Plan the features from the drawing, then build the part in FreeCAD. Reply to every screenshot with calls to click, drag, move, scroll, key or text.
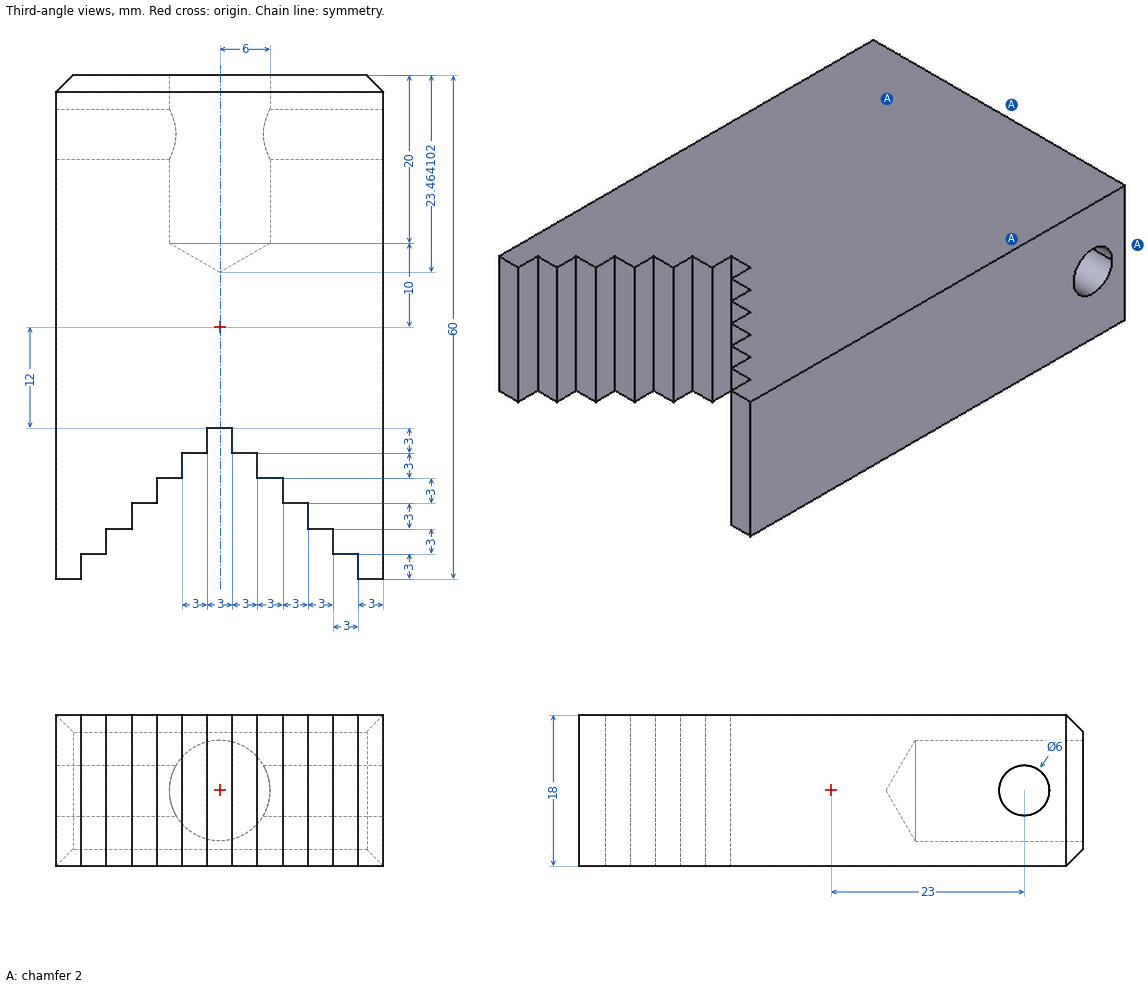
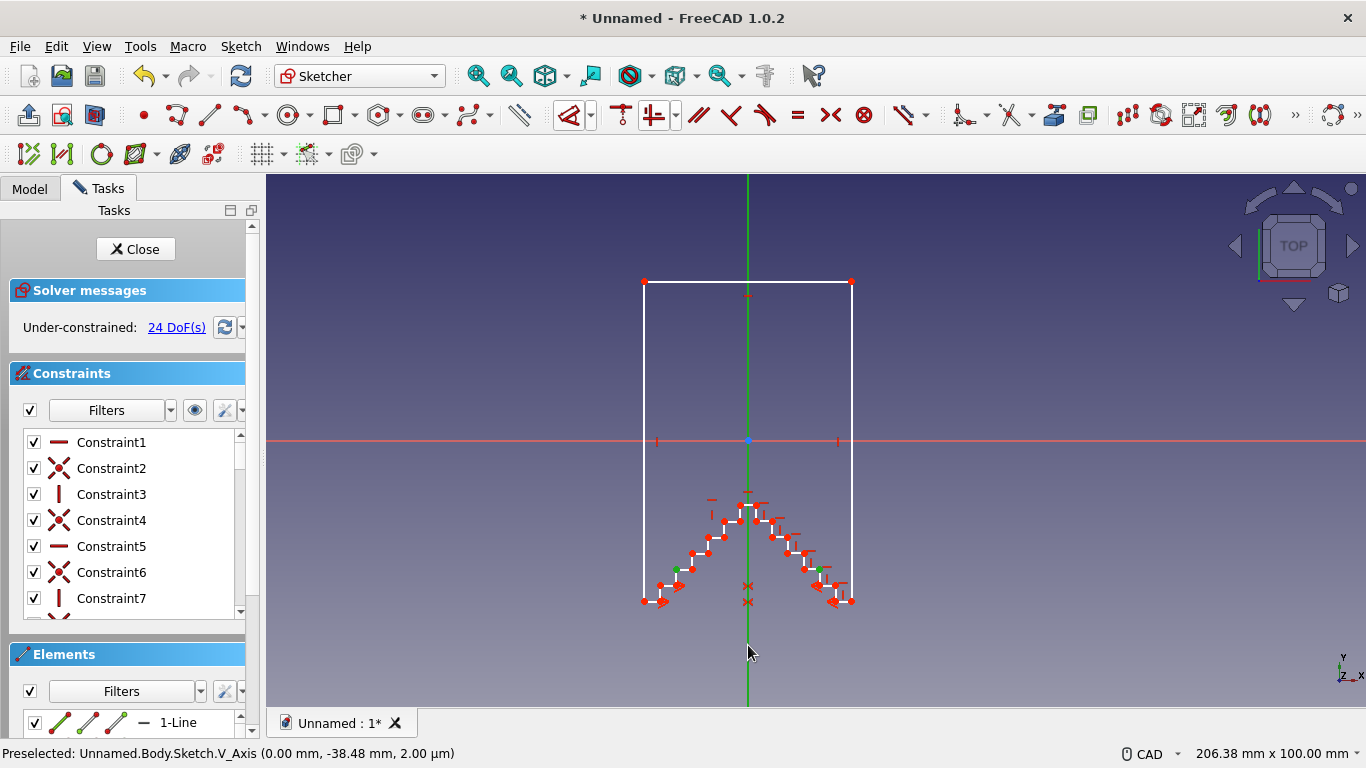
click(831, 116)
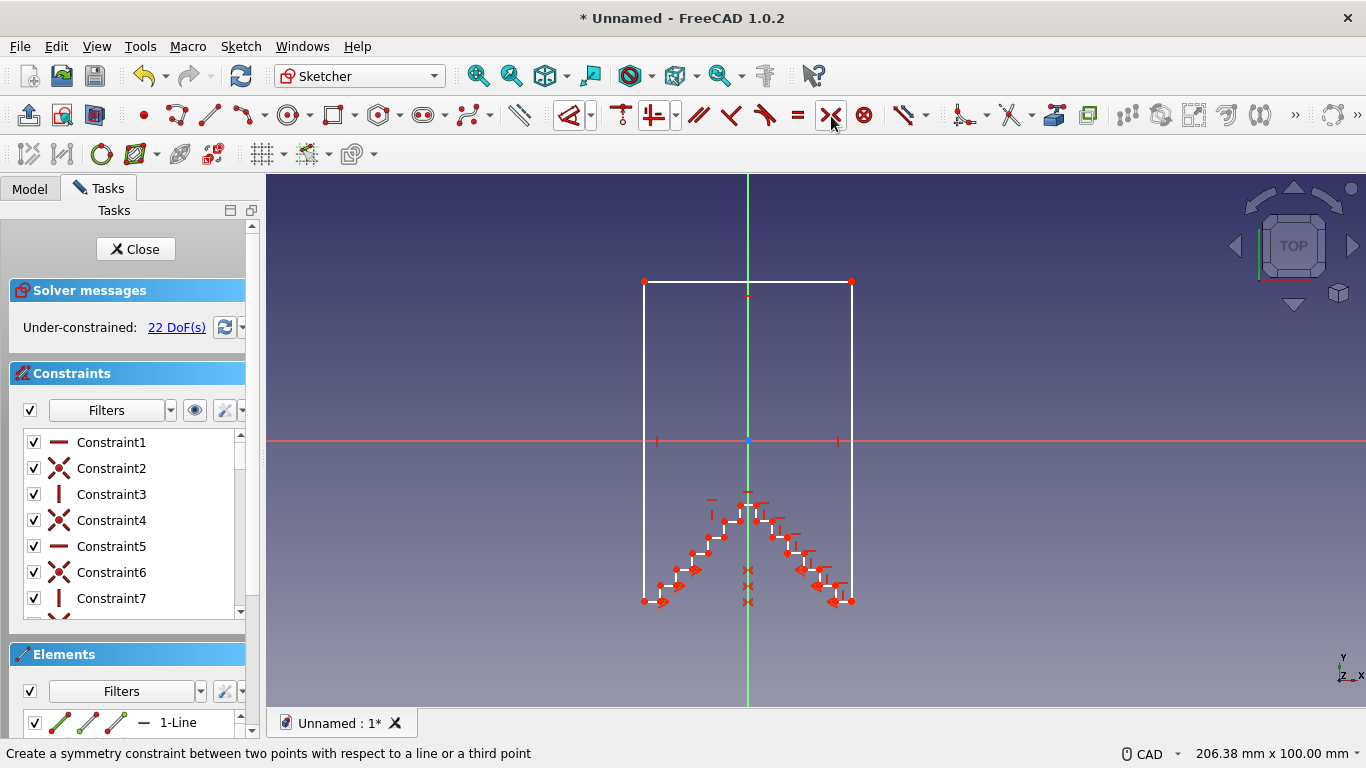
click(804, 553)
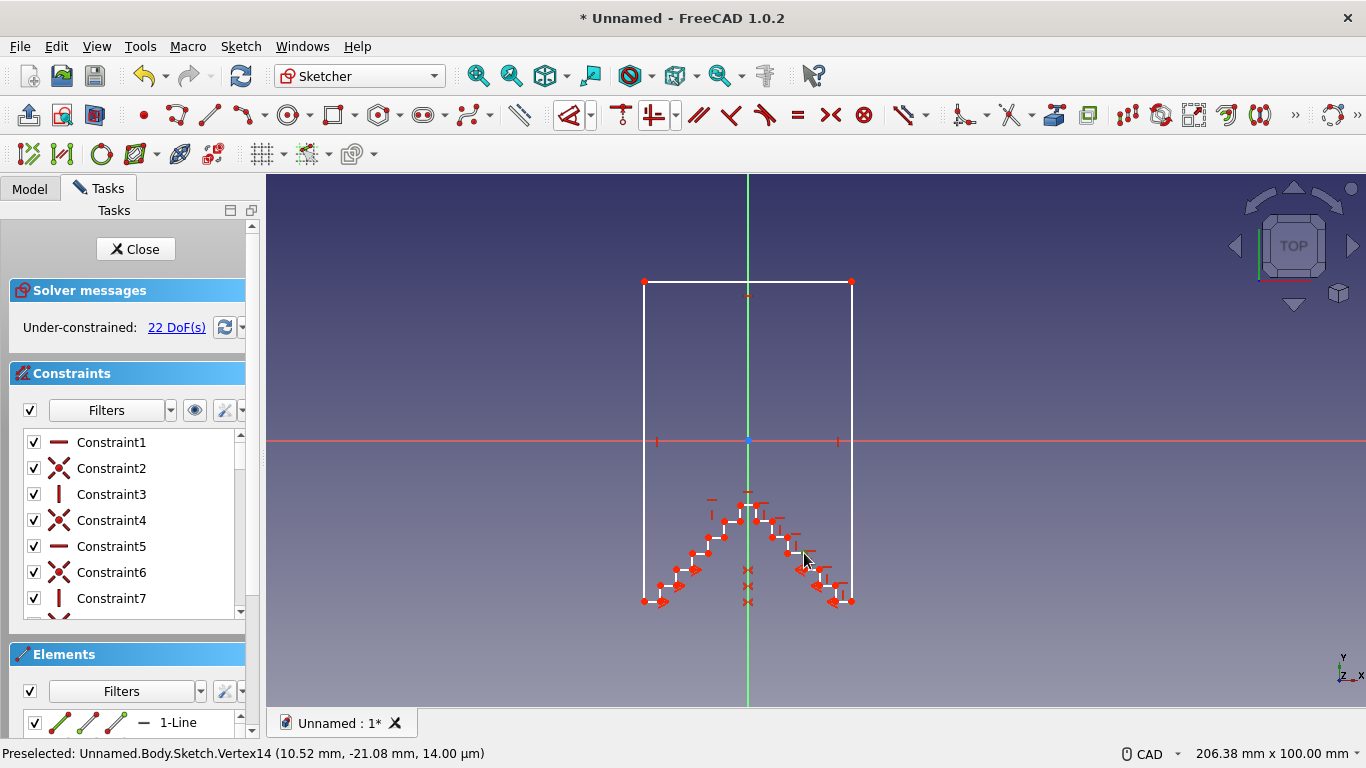
click(692, 554)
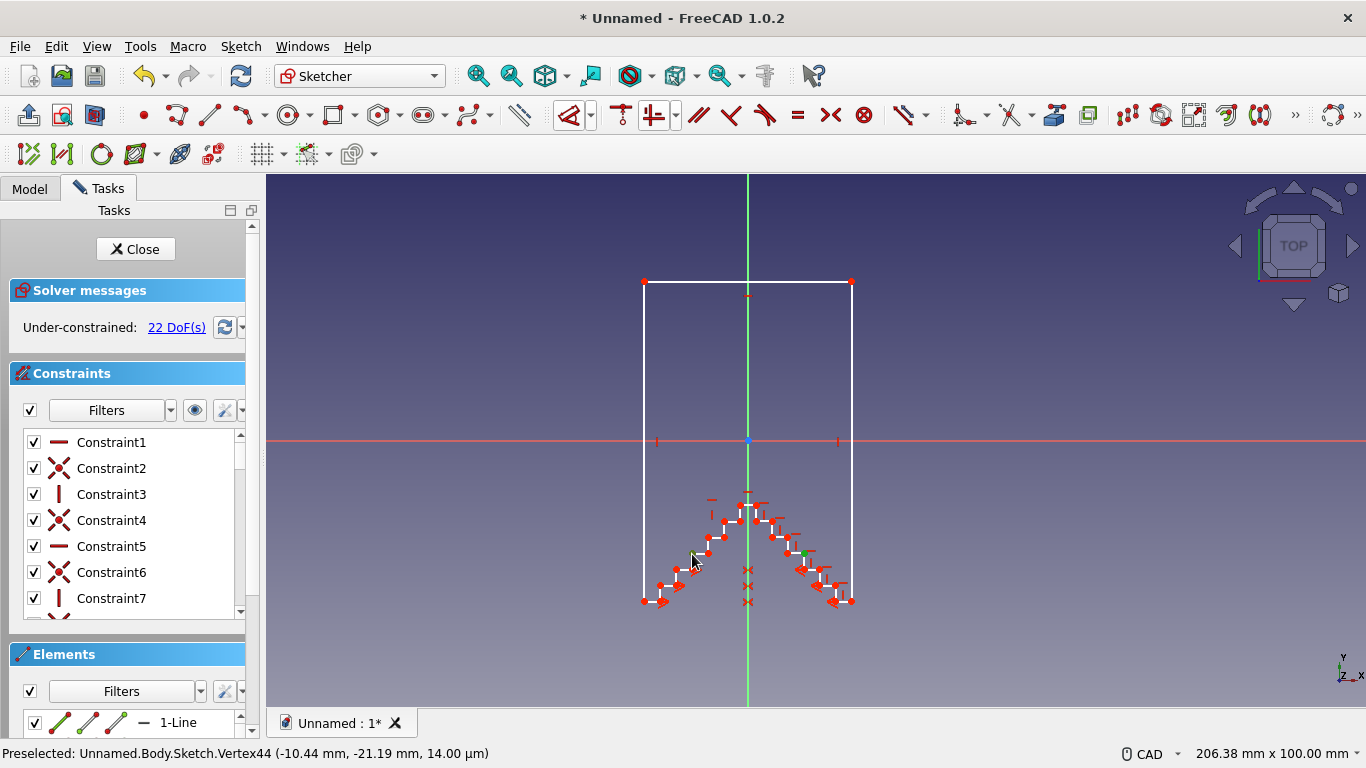
click(748, 645)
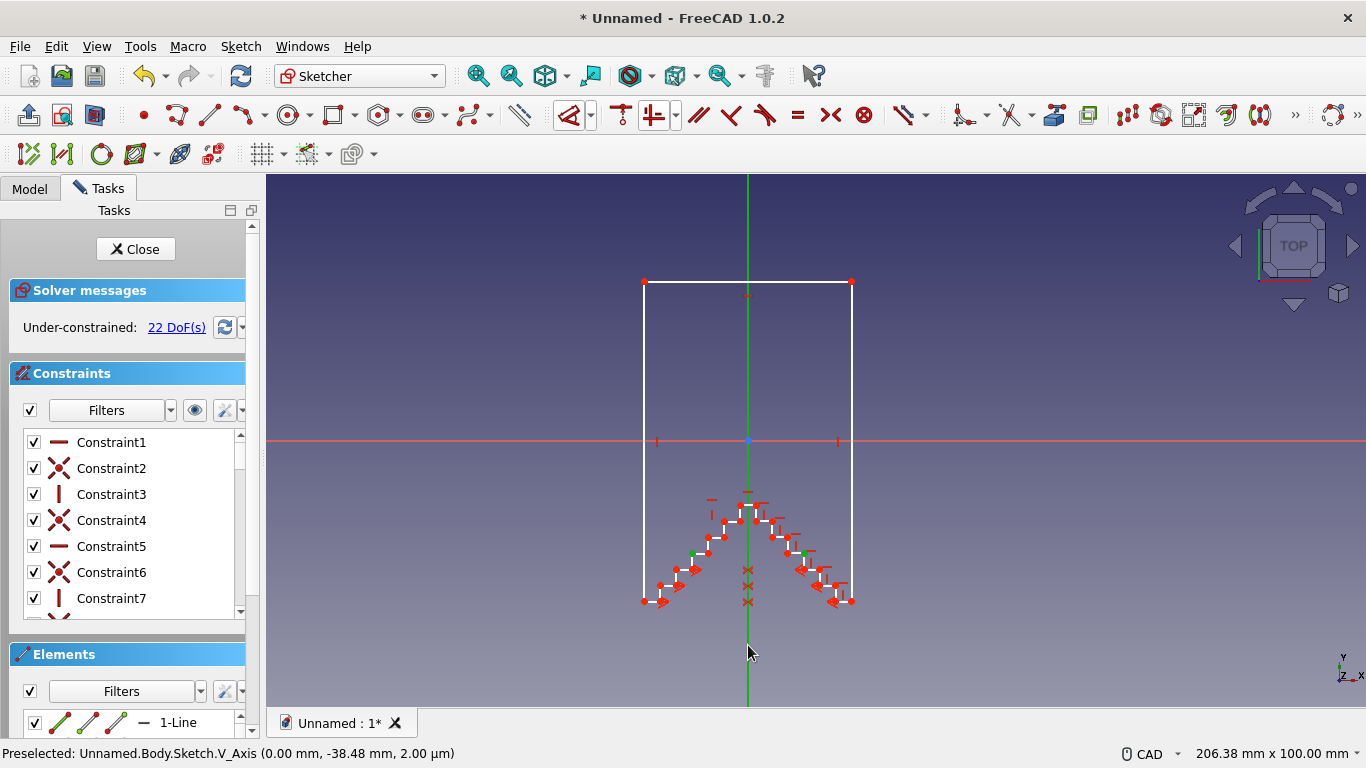
click(831, 116)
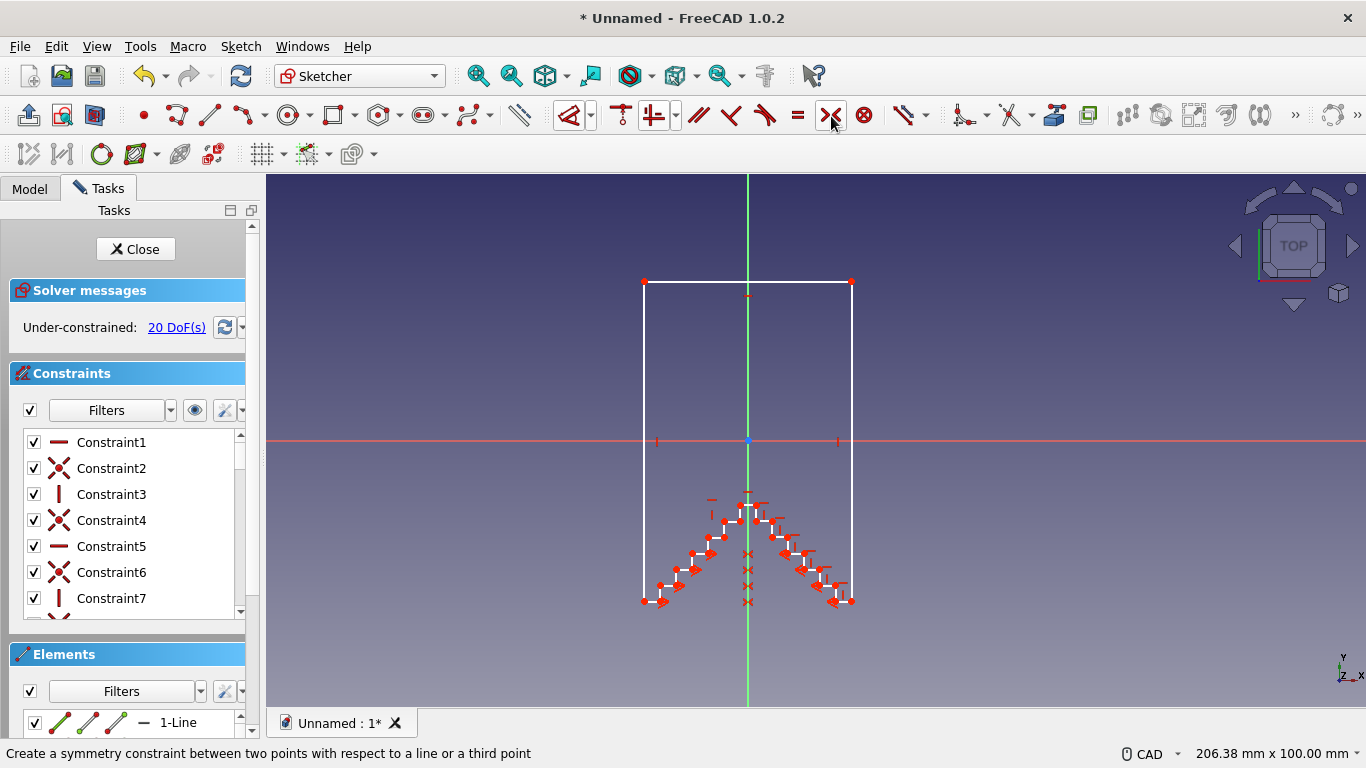
click(788, 537)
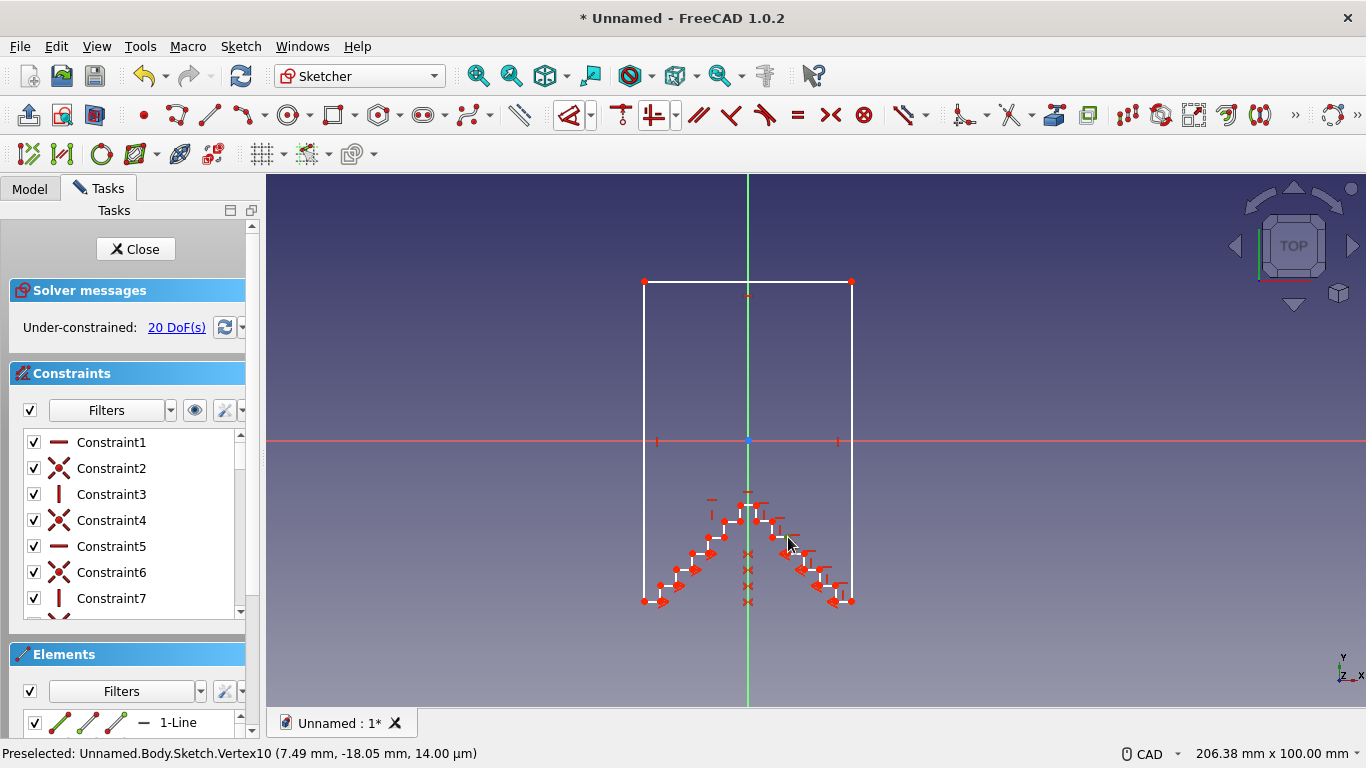
click(708, 538)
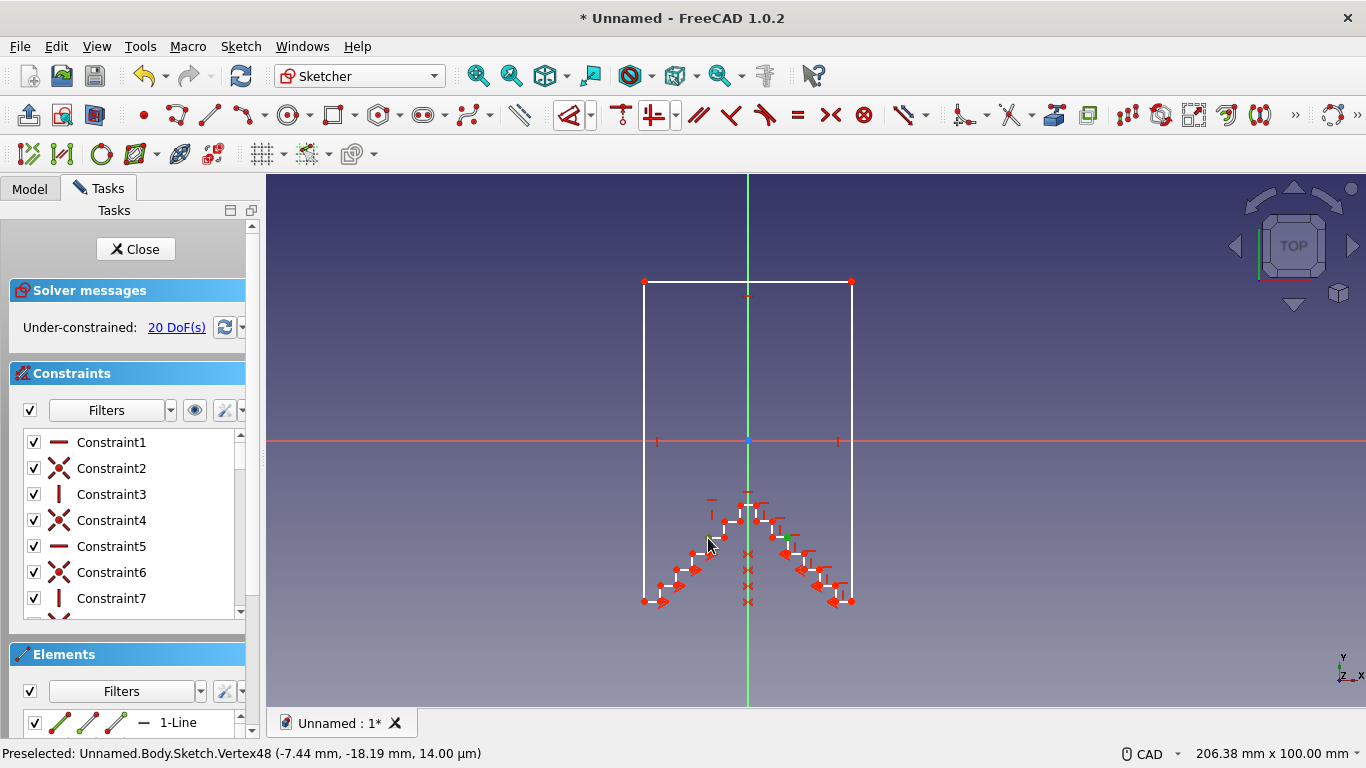
click(748, 645)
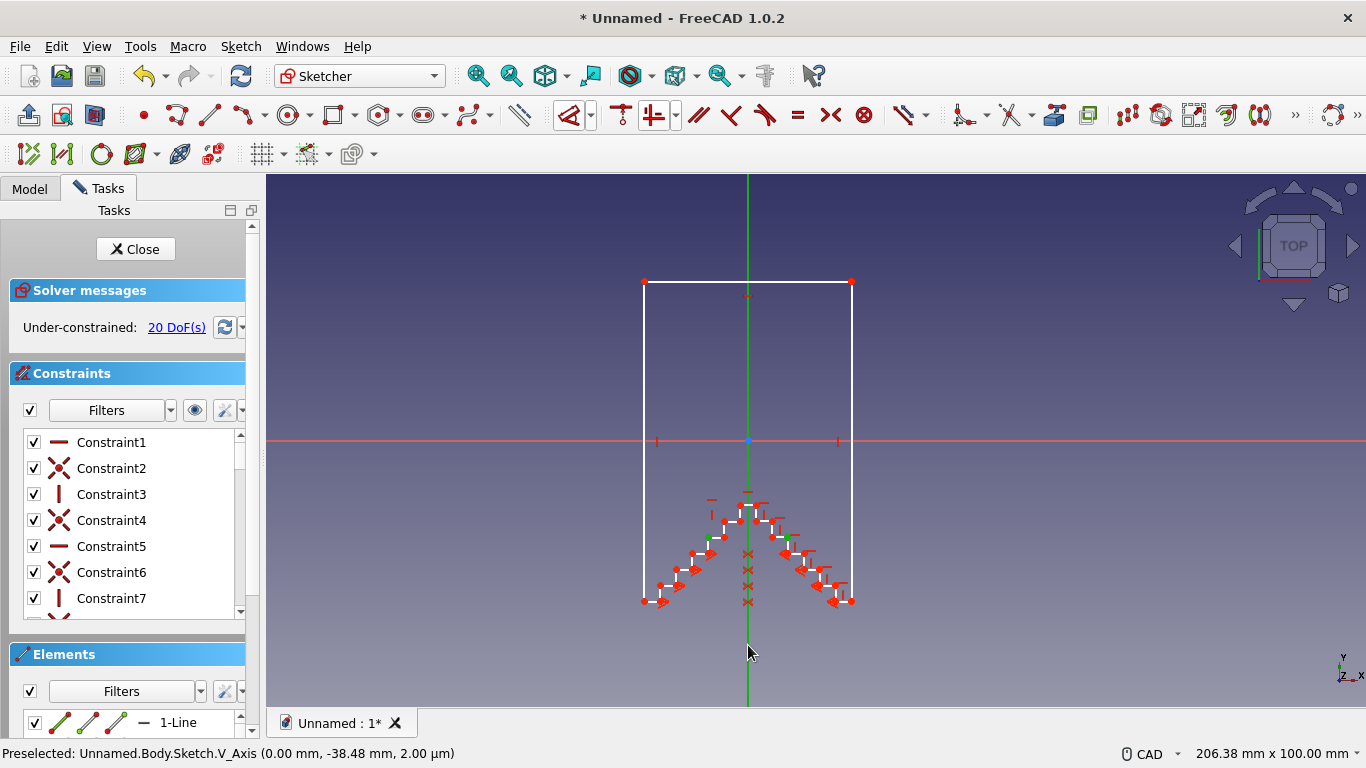
click(831, 116)